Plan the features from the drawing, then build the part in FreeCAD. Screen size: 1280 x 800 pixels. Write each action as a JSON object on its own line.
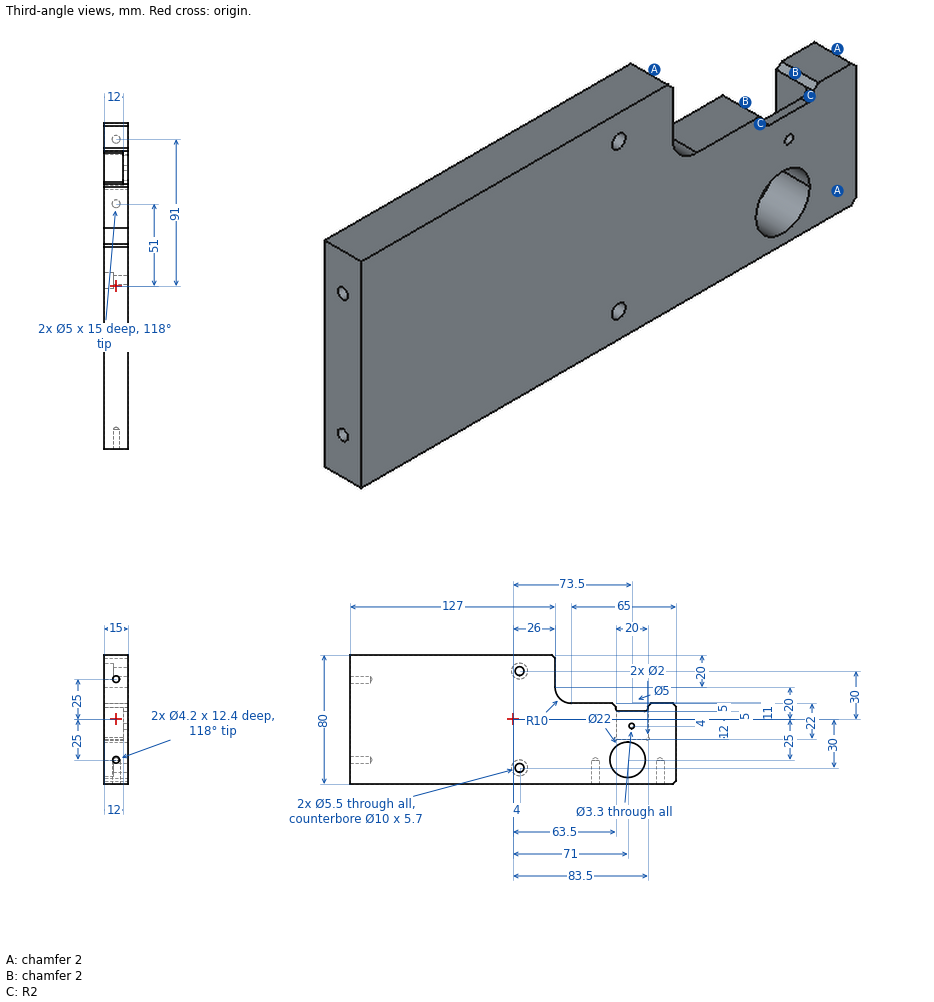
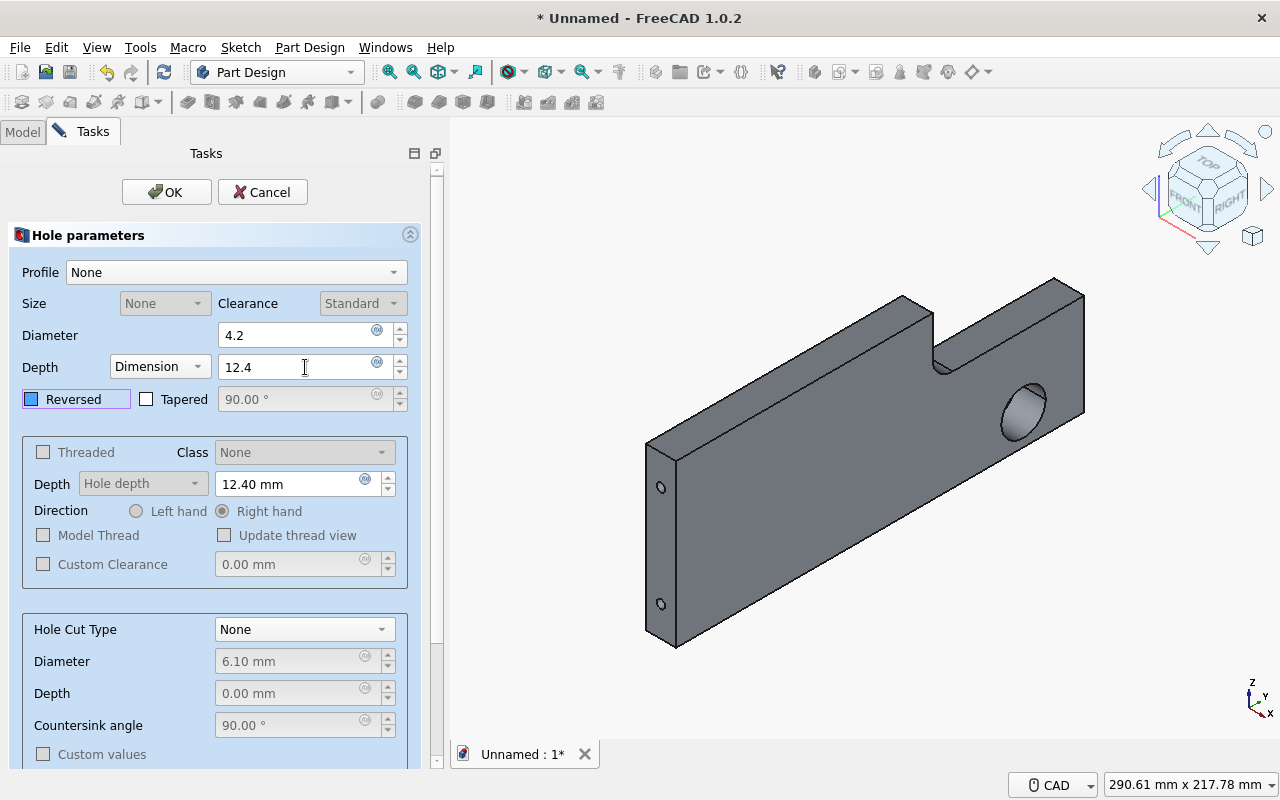
{"action": "left_click", "coordinate": [167, 192]}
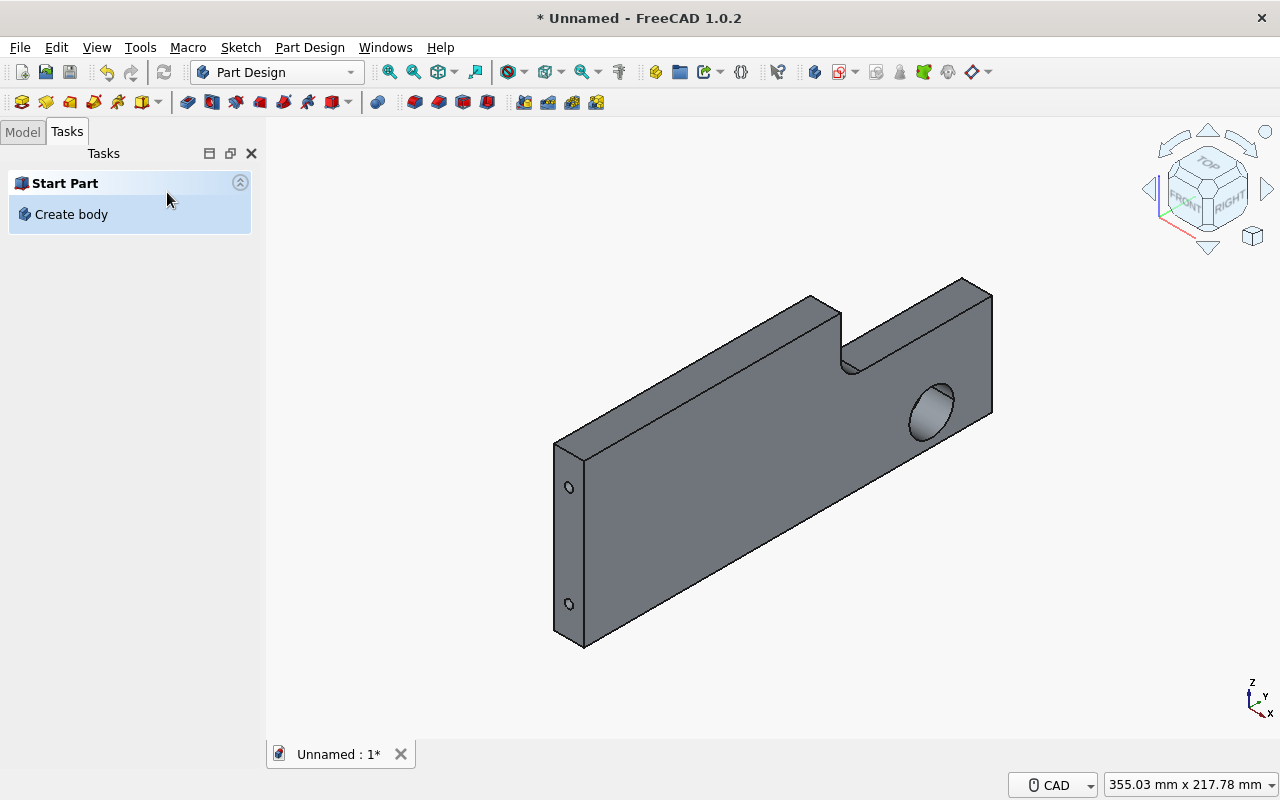
{"action": "key", "text": "6"}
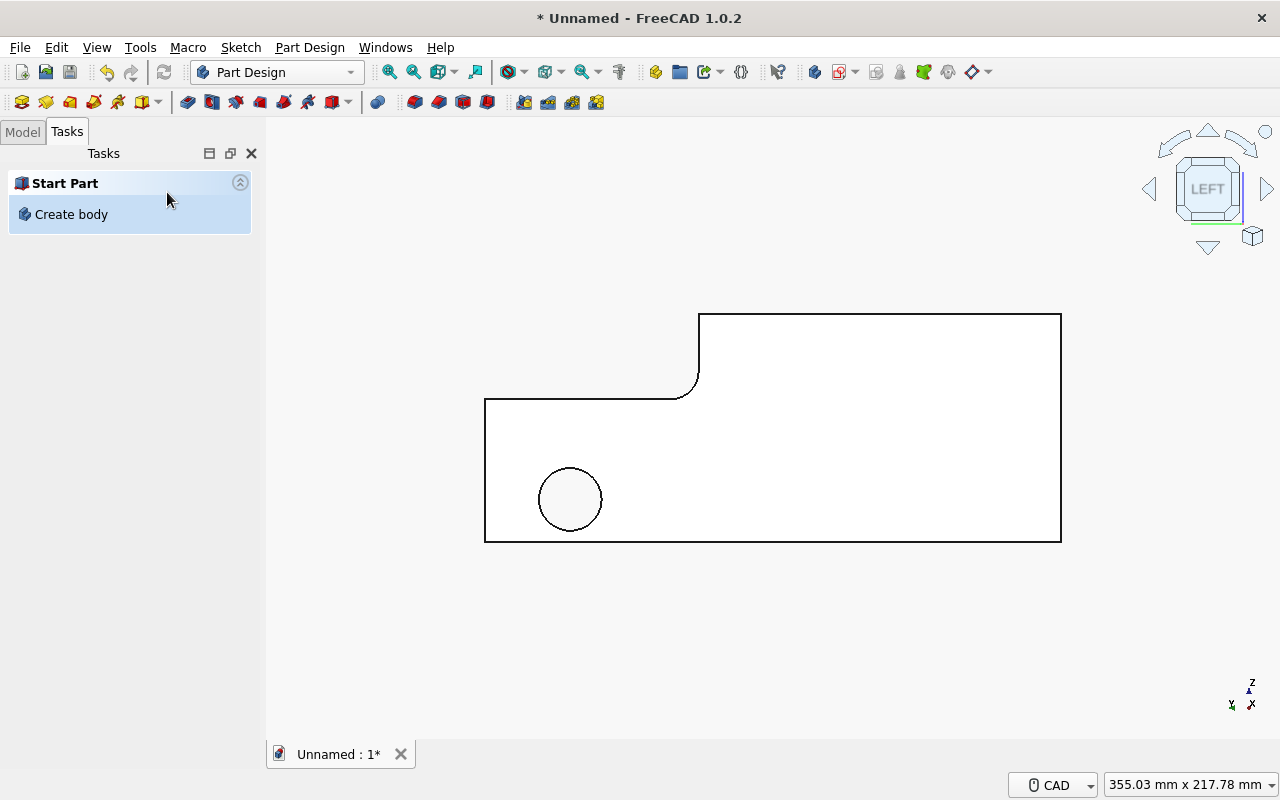
{"action": "left_click", "coordinate": [855, 427]}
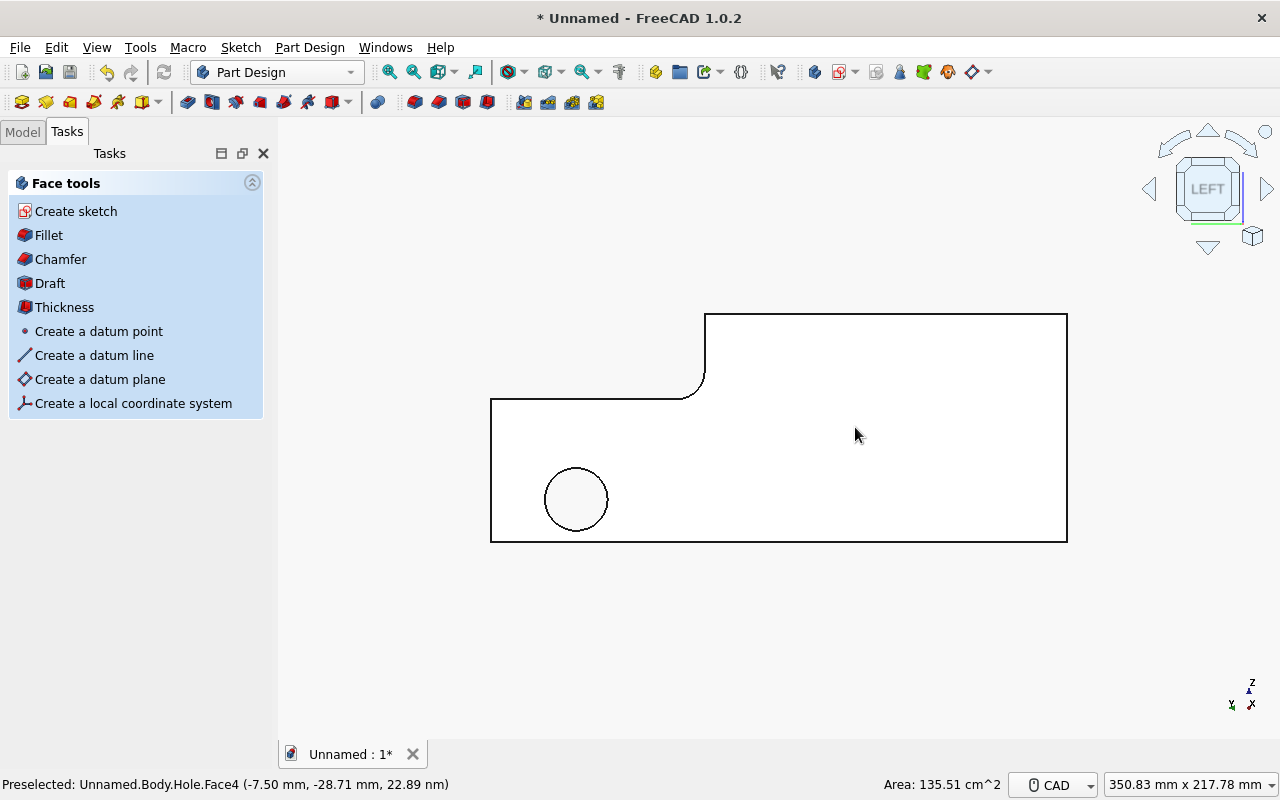
{"action": "left_click", "coordinate": [840, 72]}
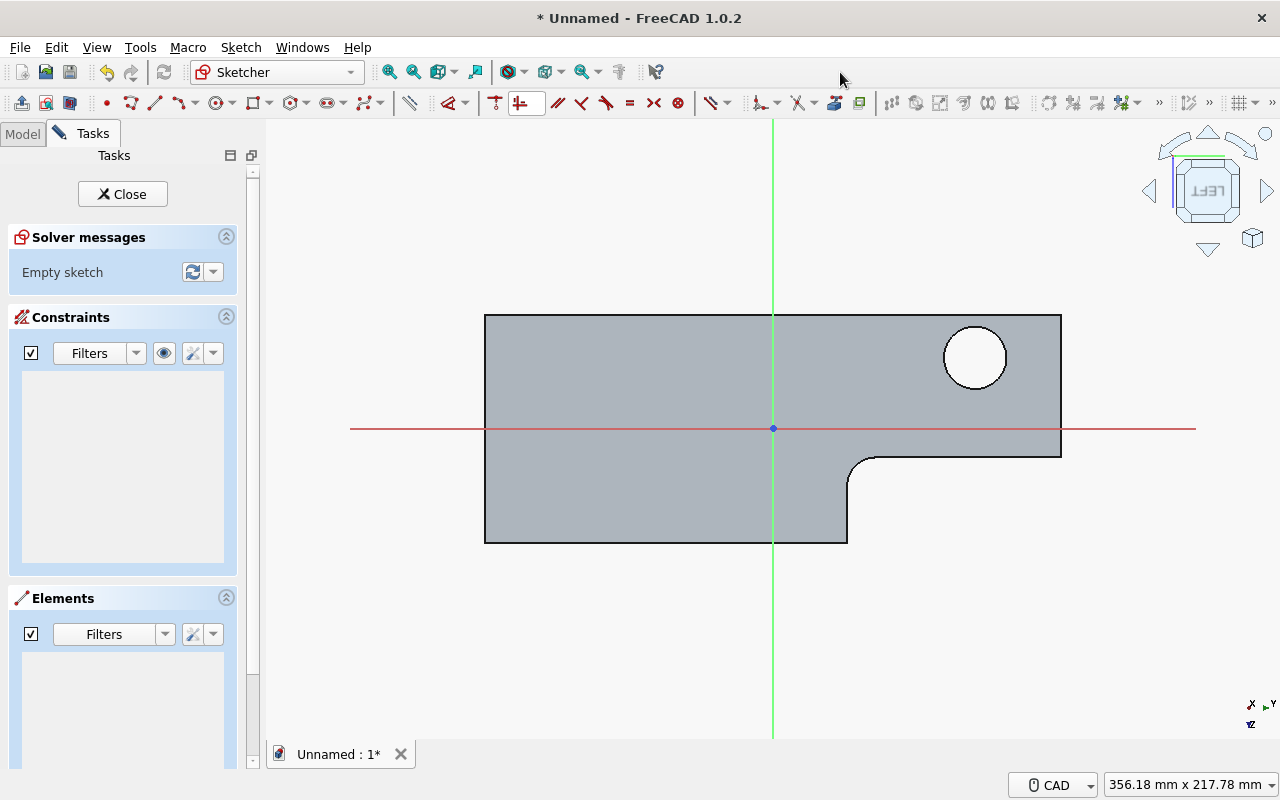
{"action": "scroll", "coordinate": [846, 429], "scroll_direction": "up", "scroll_amount": 4}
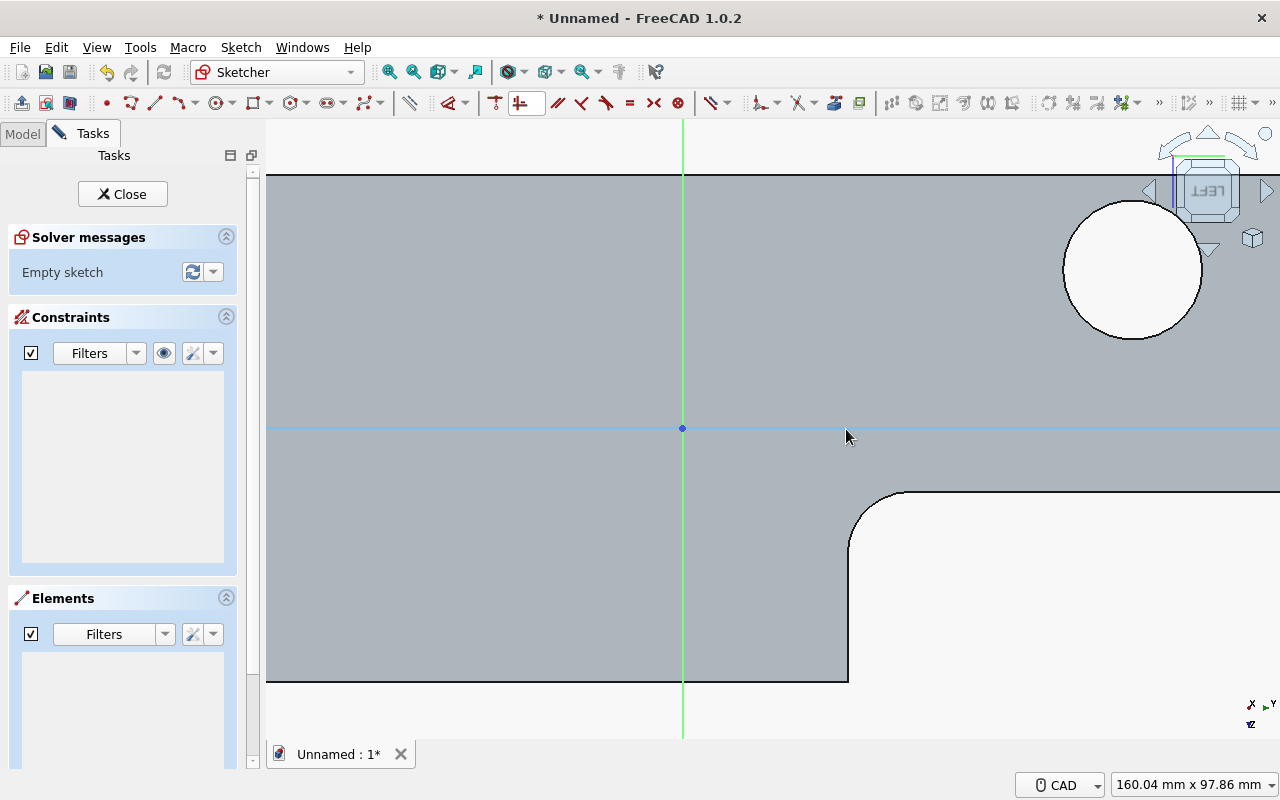
{"action": "left_click", "coordinate": [216, 104]}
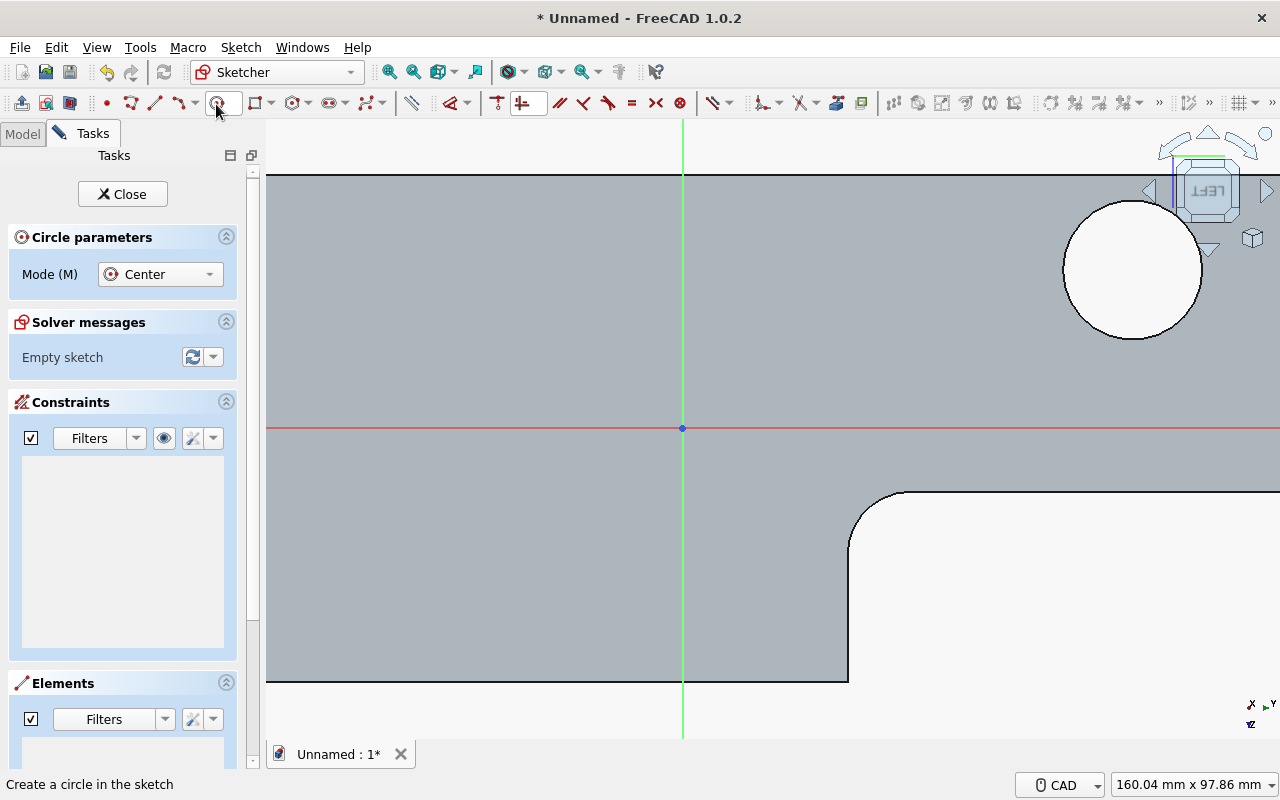
{"action": "scroll", "coordinate": [708, 238], "scroll_direction": "up", "scroll_amount": 2}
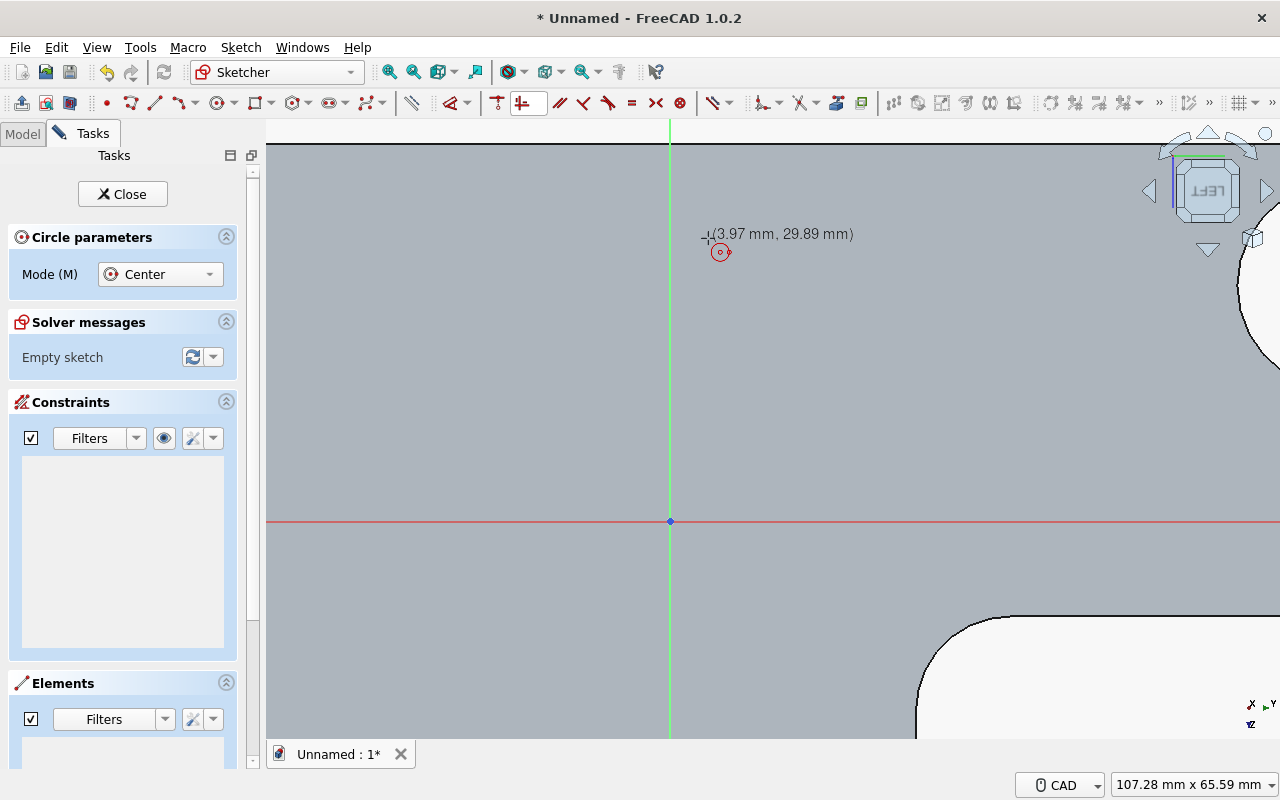
{"action": "left_click", "coordinate": [708, 238]}
{"action": "left_click", "coordinate": [726, 220]}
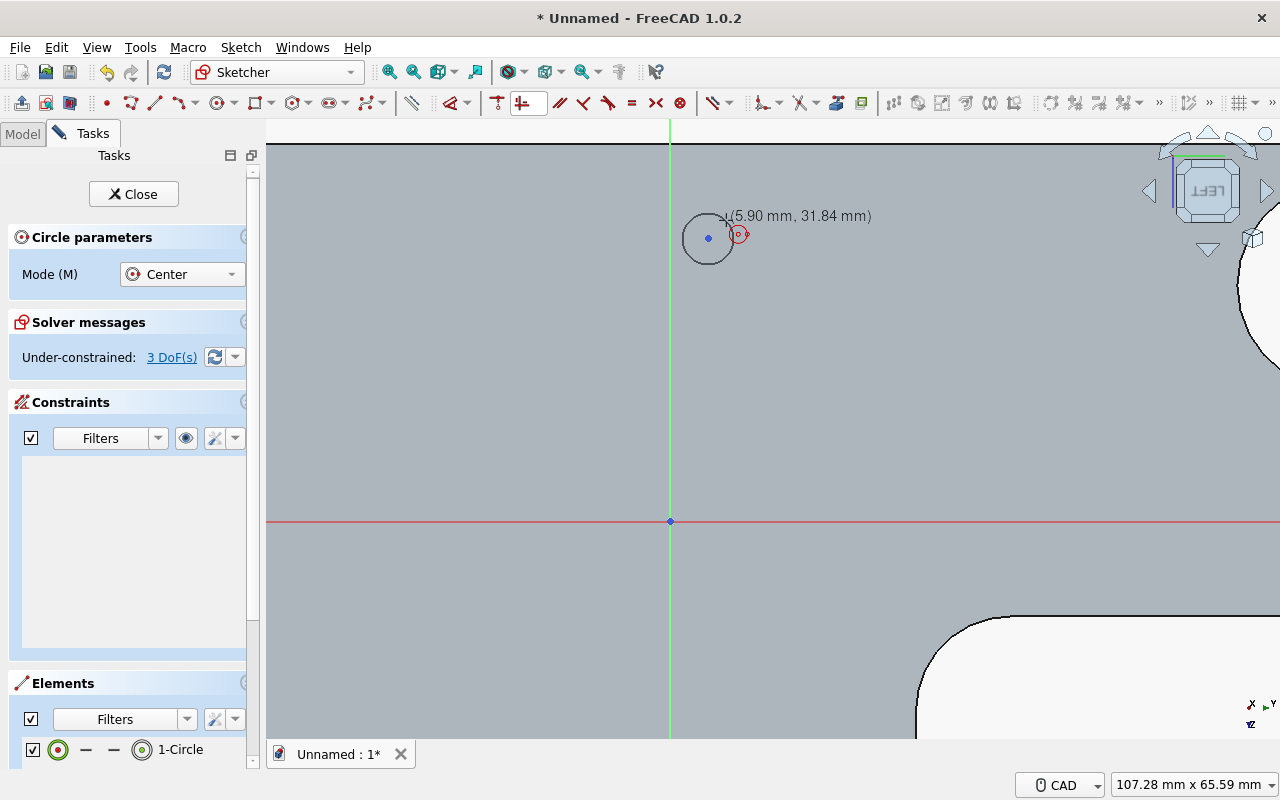
{"action": "scroll", "coordinate": [709, 240], "scroll_direction": "down", "scroll_amount": 2}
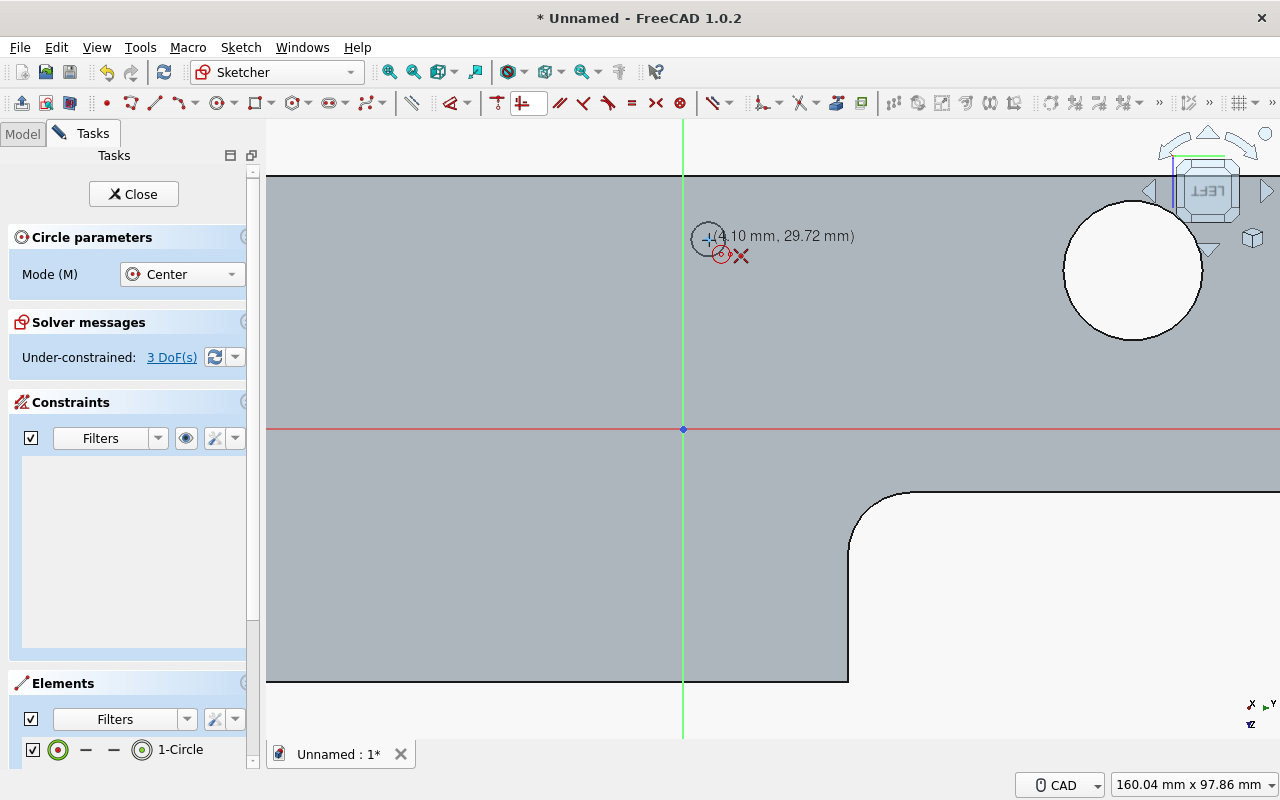
{"action": "scroll", "coordinate": [709, 619], "scroll_direction": "up", "scroll_amount": 2}